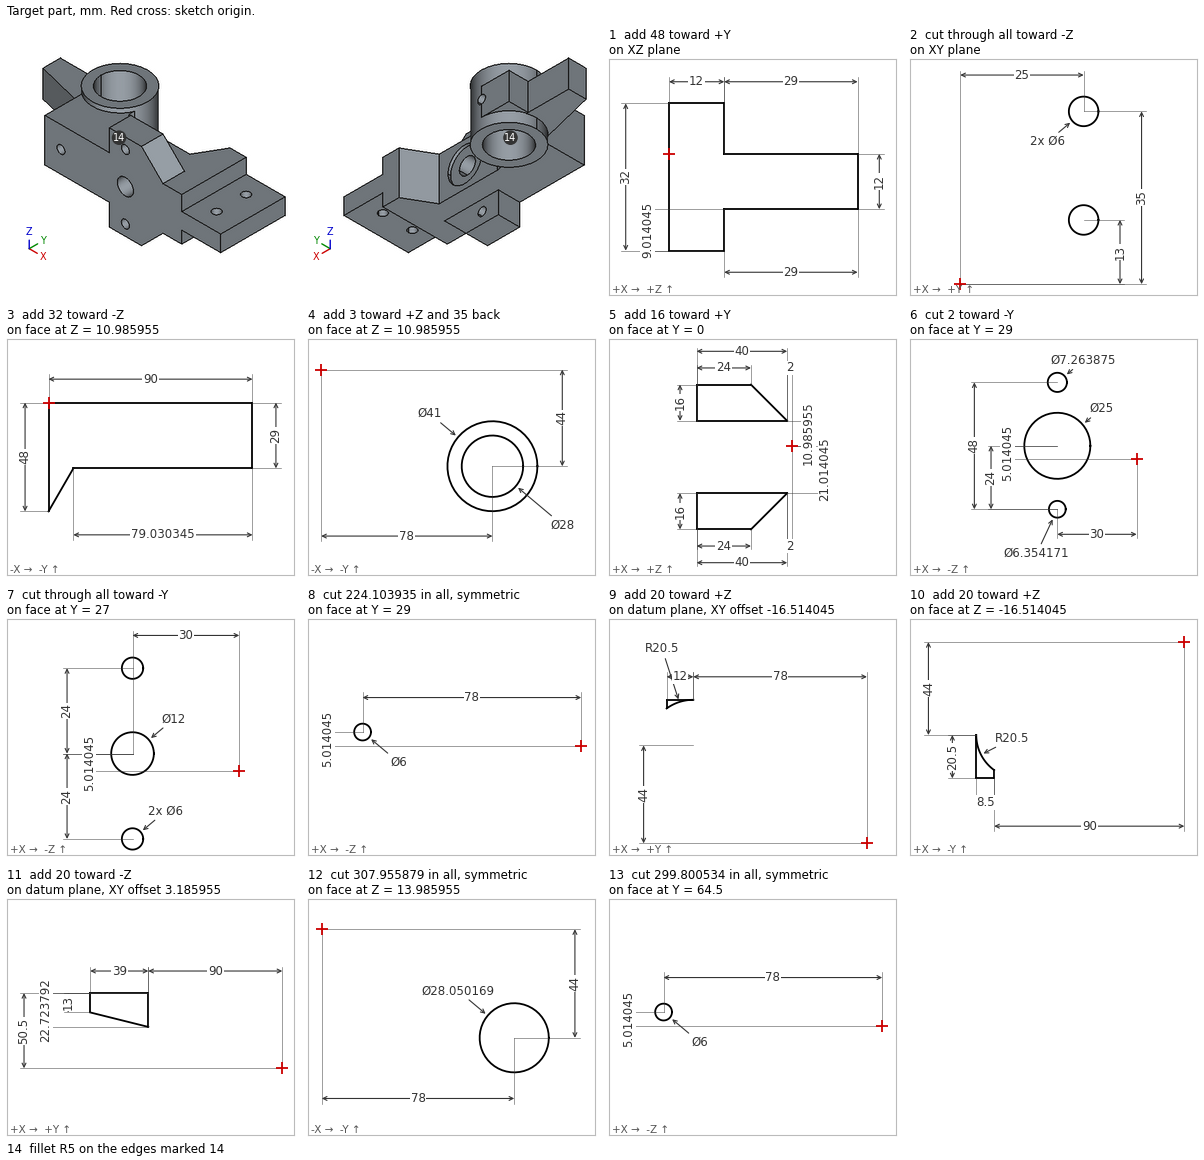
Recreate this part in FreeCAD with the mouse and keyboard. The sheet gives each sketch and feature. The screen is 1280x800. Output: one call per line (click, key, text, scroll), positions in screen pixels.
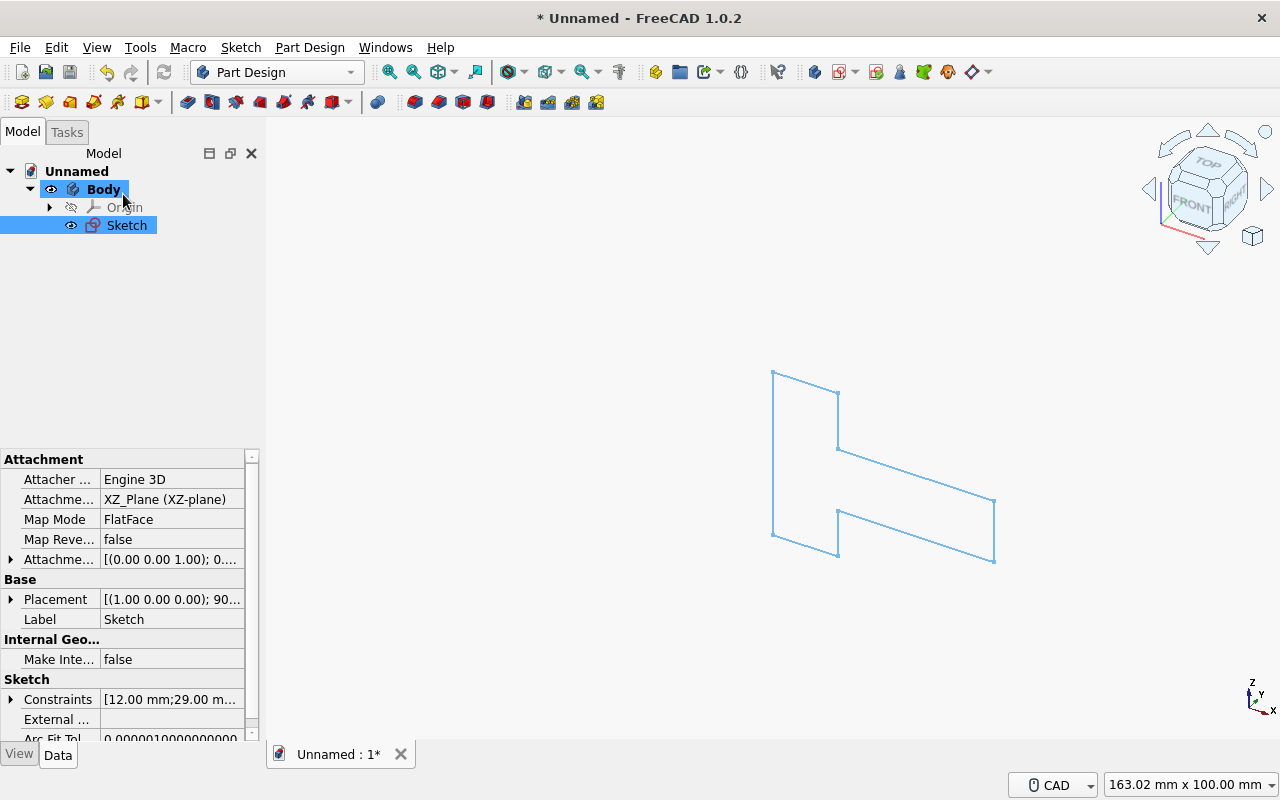
click(22, 102)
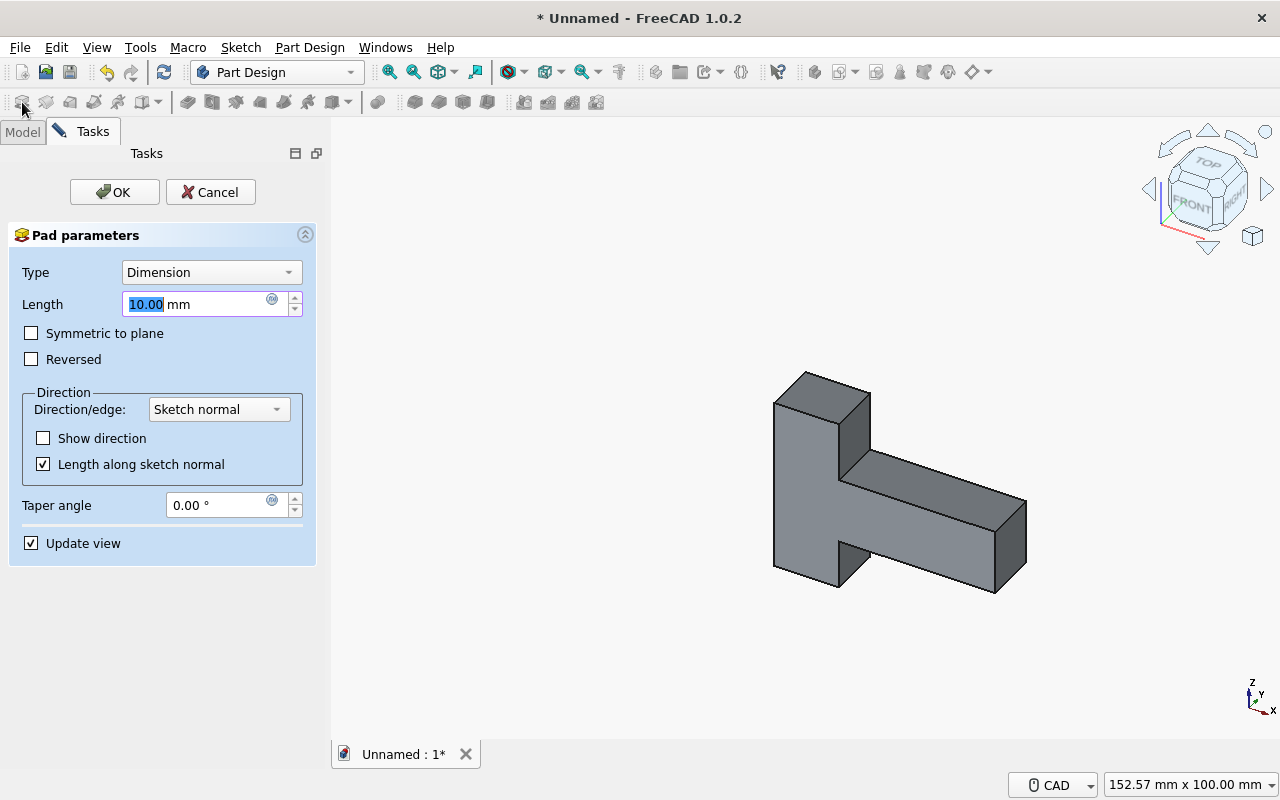
text(48)
key(Tab)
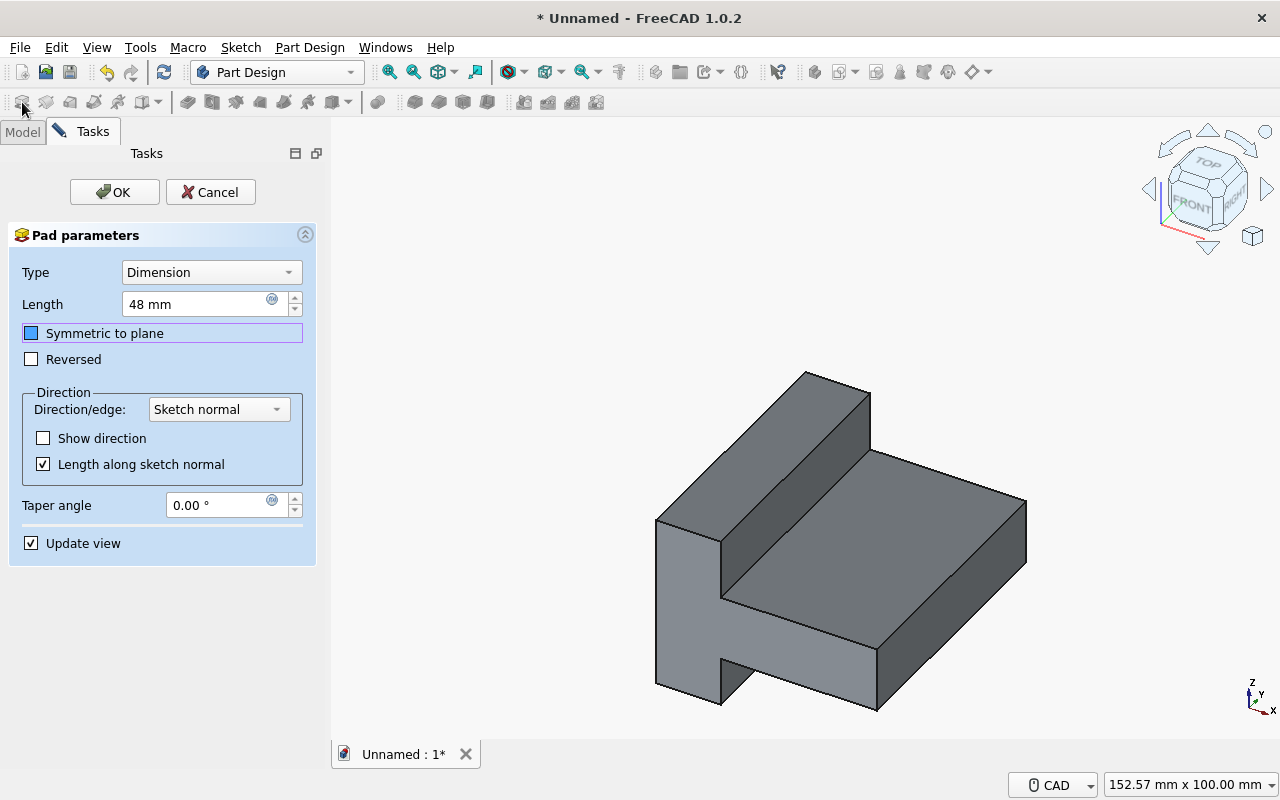
click(30, 359)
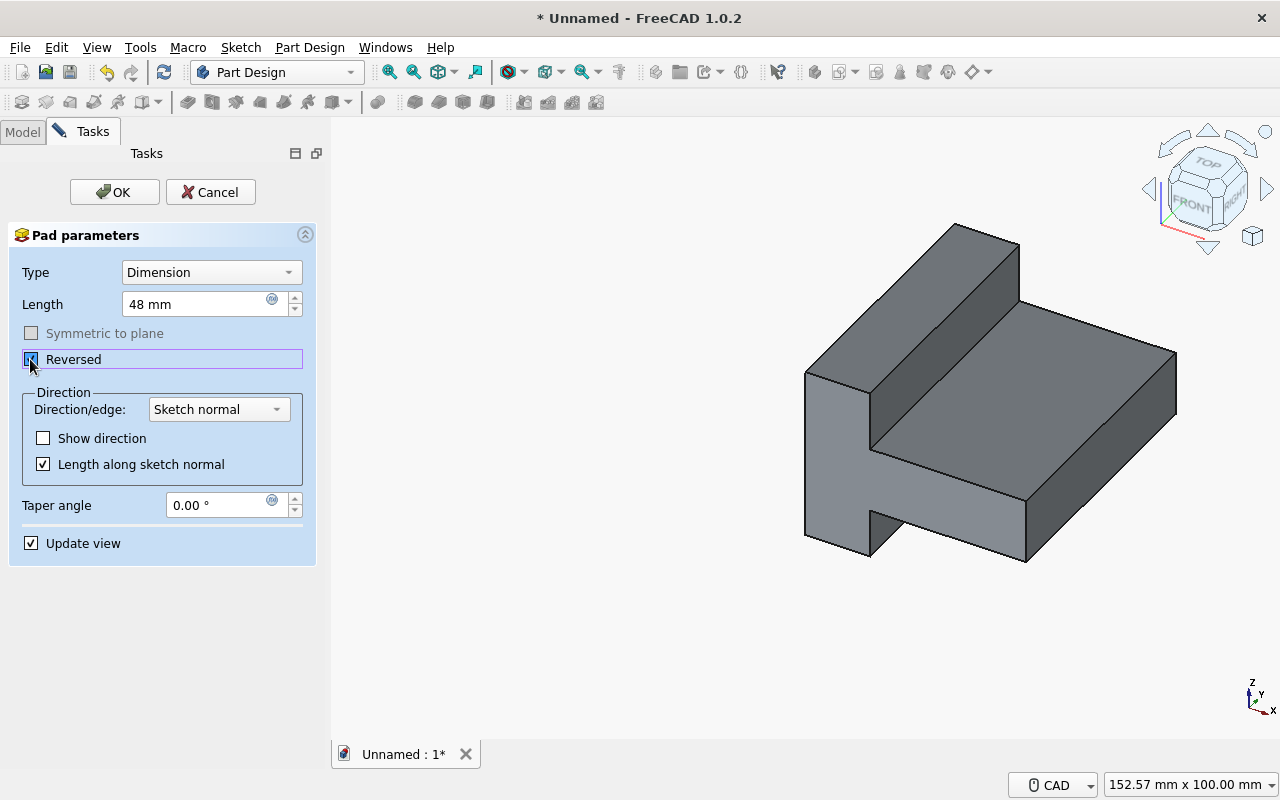
click(115, 192)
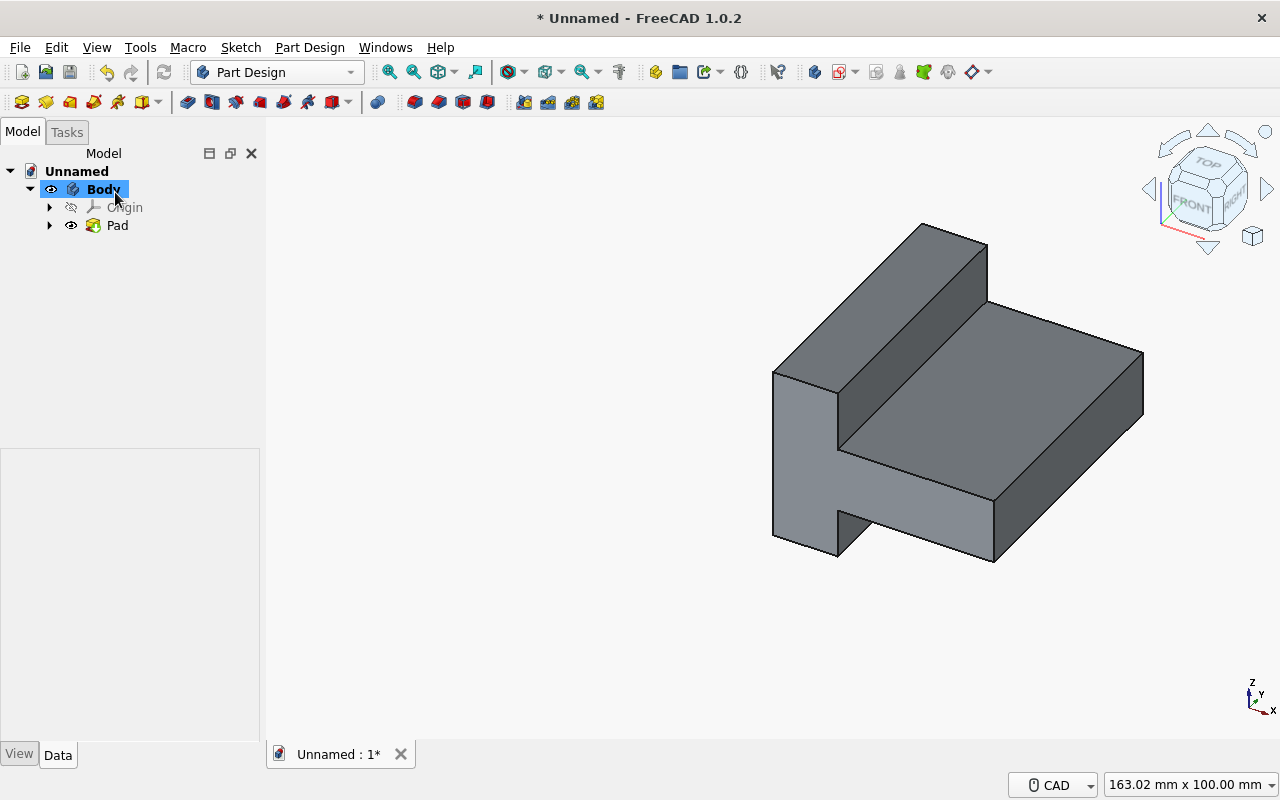
click(840, 72)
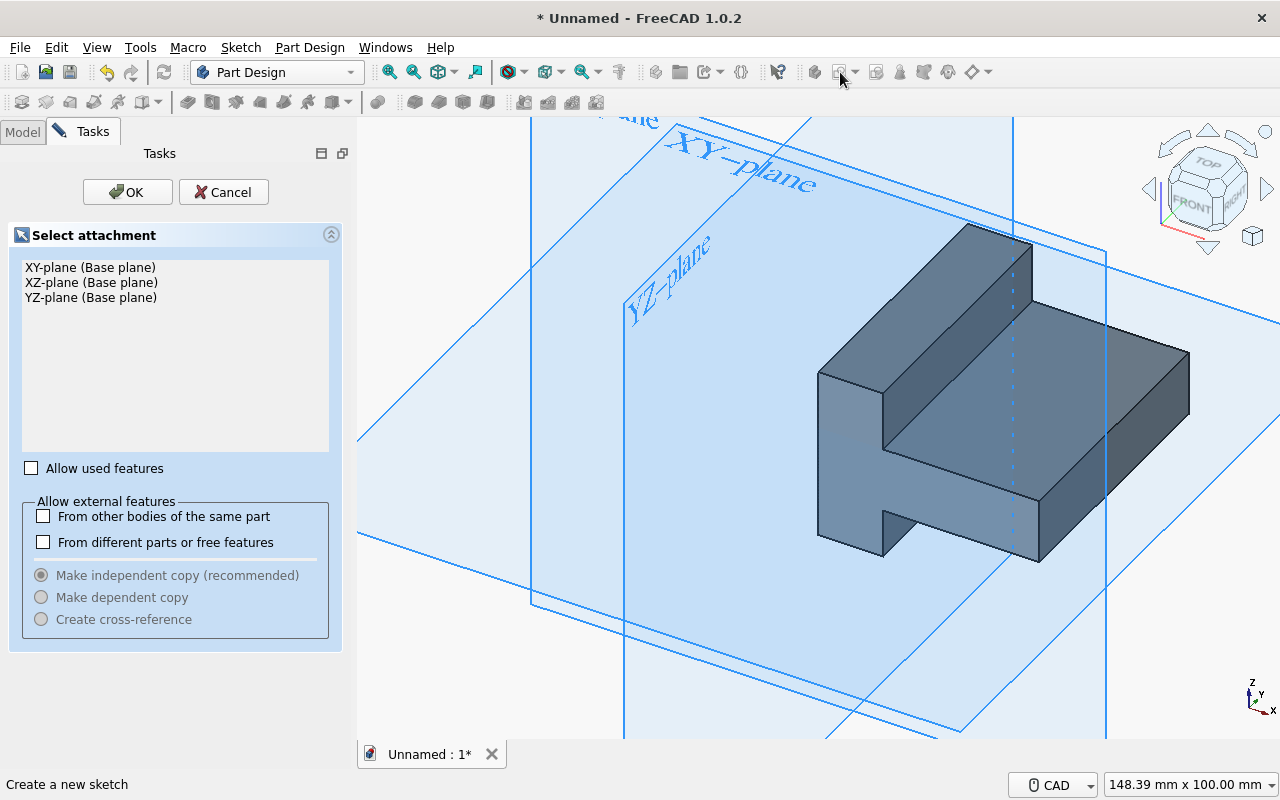
click(82, 268)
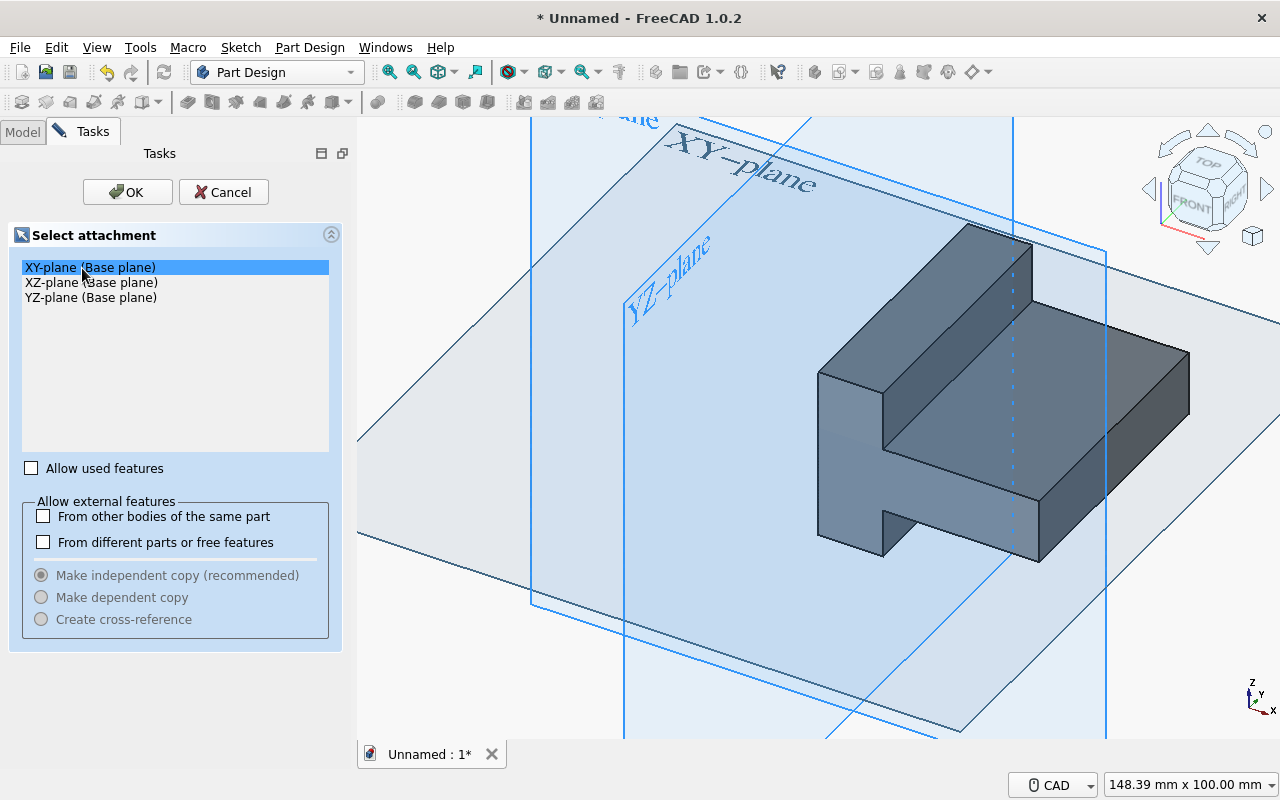
click(128, 192)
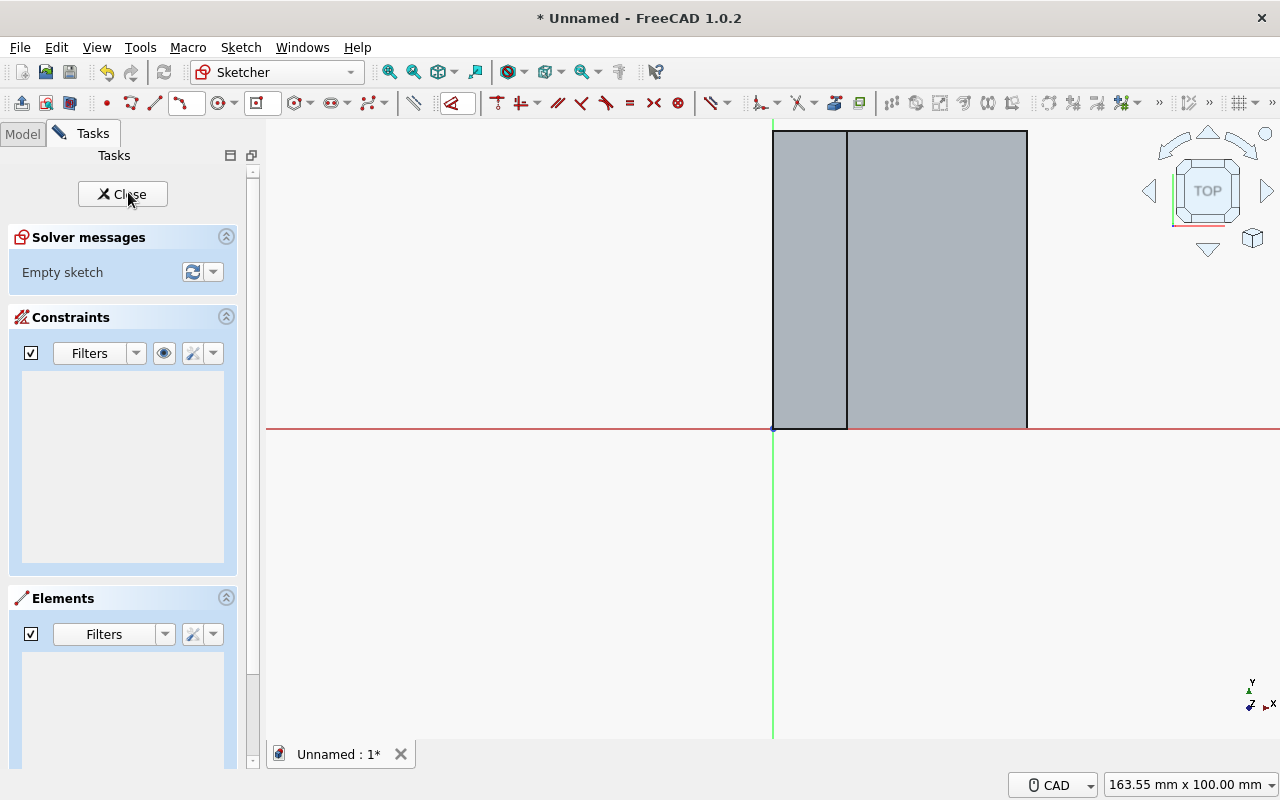
click(70, 104)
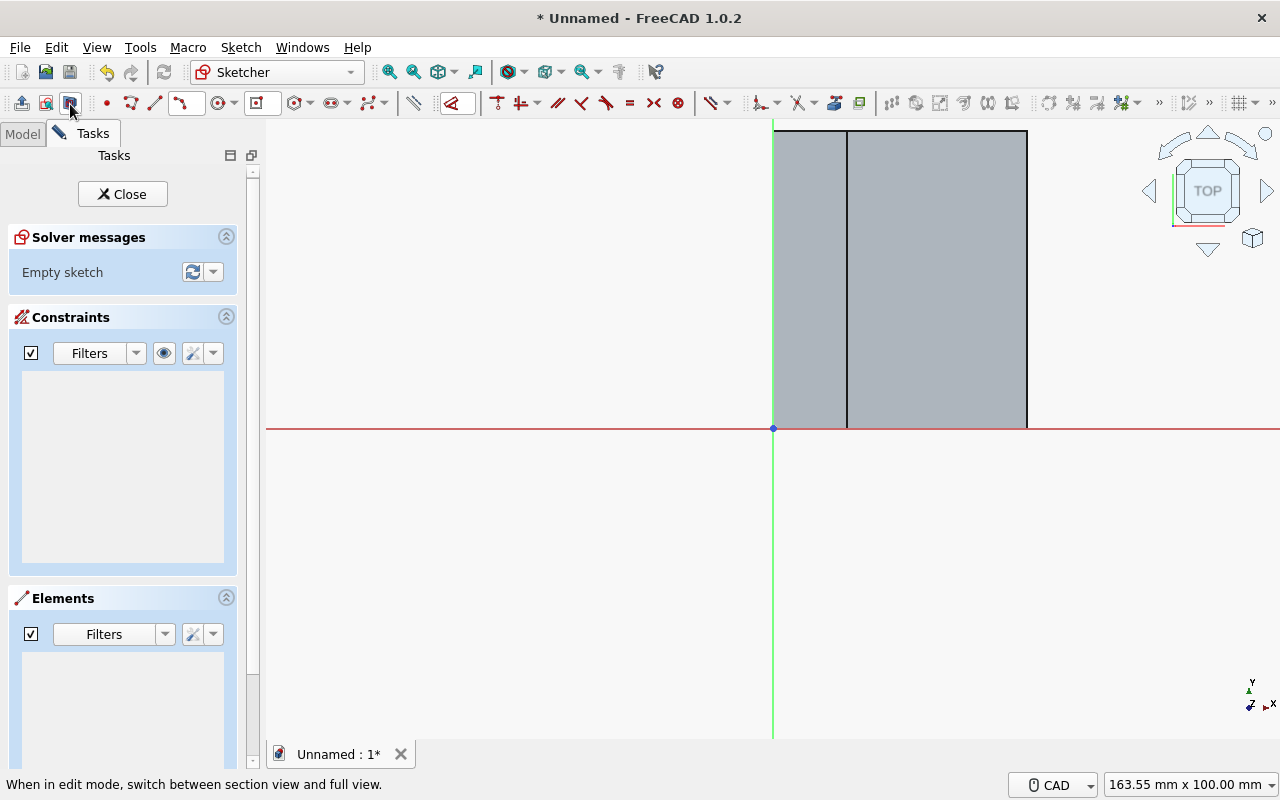
scroll(1049, 168, up, 3)